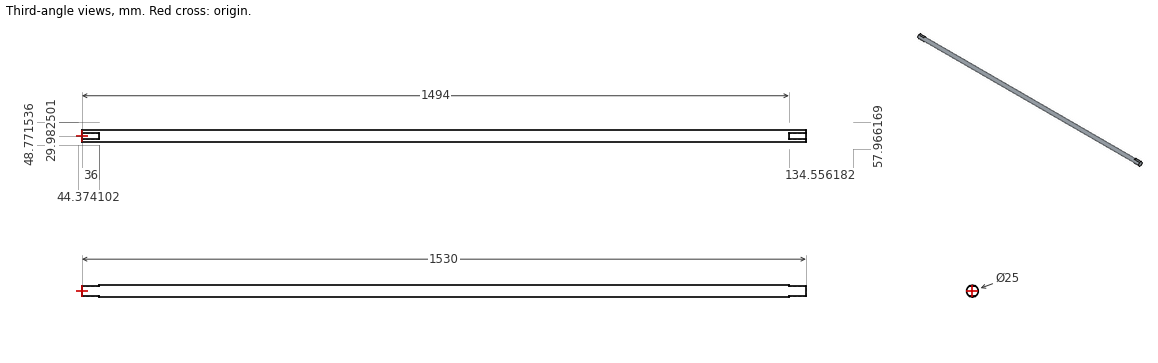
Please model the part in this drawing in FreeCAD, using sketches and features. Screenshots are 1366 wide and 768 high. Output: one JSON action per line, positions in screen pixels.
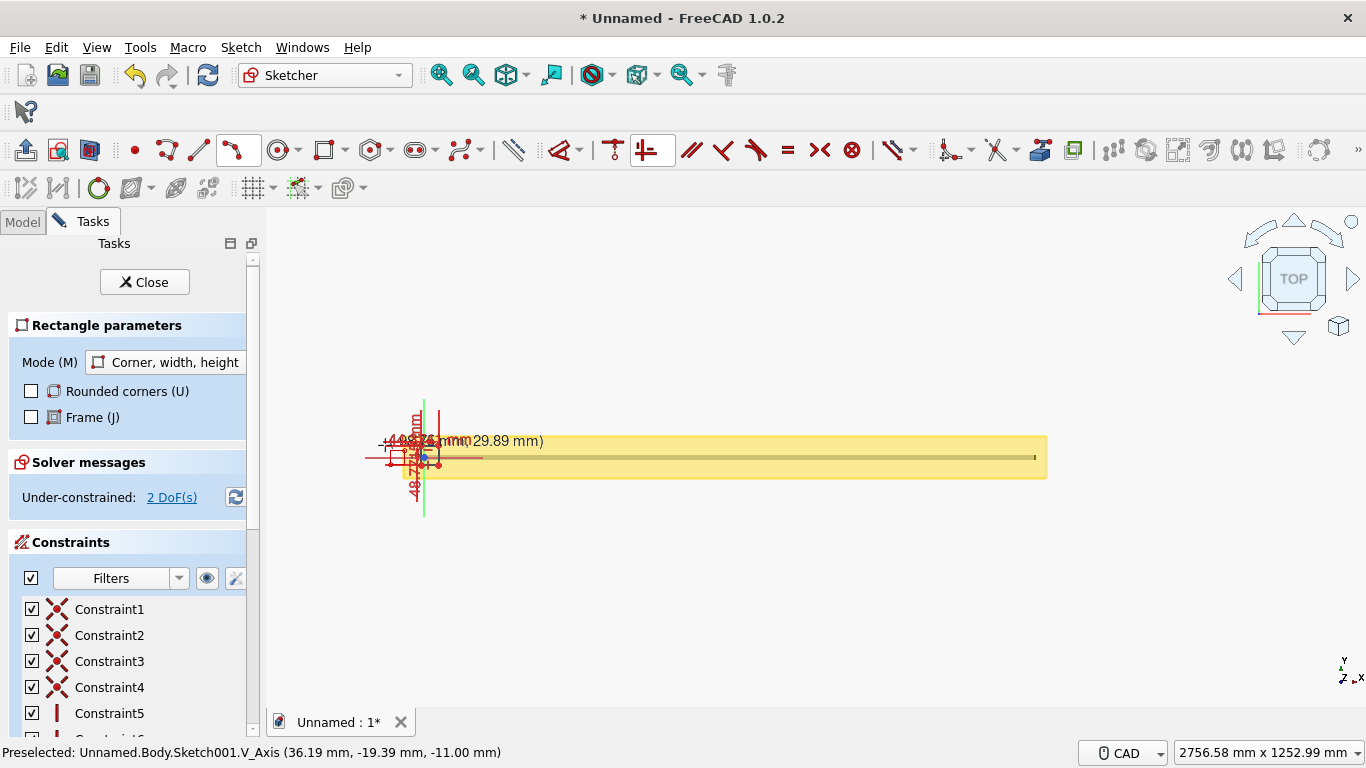
{"action": "scroll", "coordinate": [1021, 446], "scroll_direction": "up", "scroll_amount": 2}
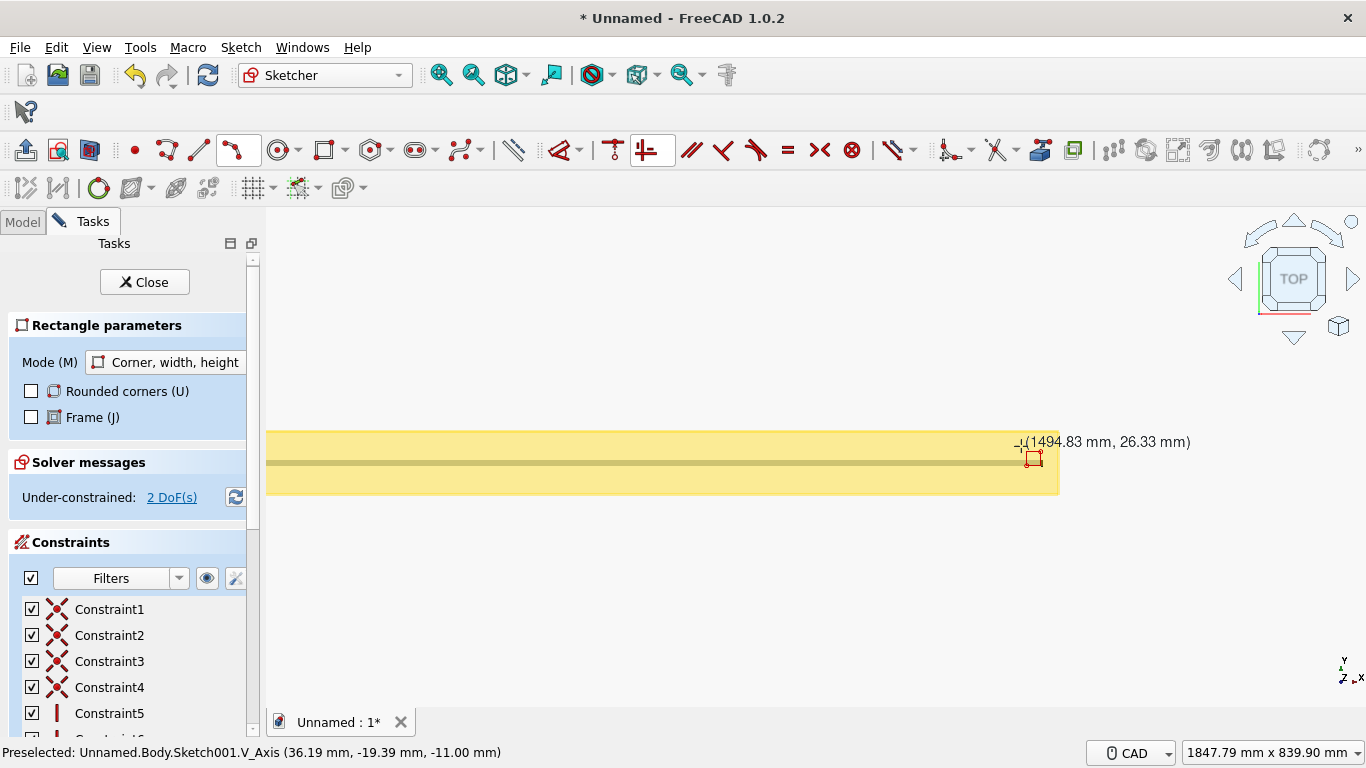
{"action": "left_click", "coordinate": [1020, 445]}
{"action": "mouse_move", "coordinate": [1100, 480]}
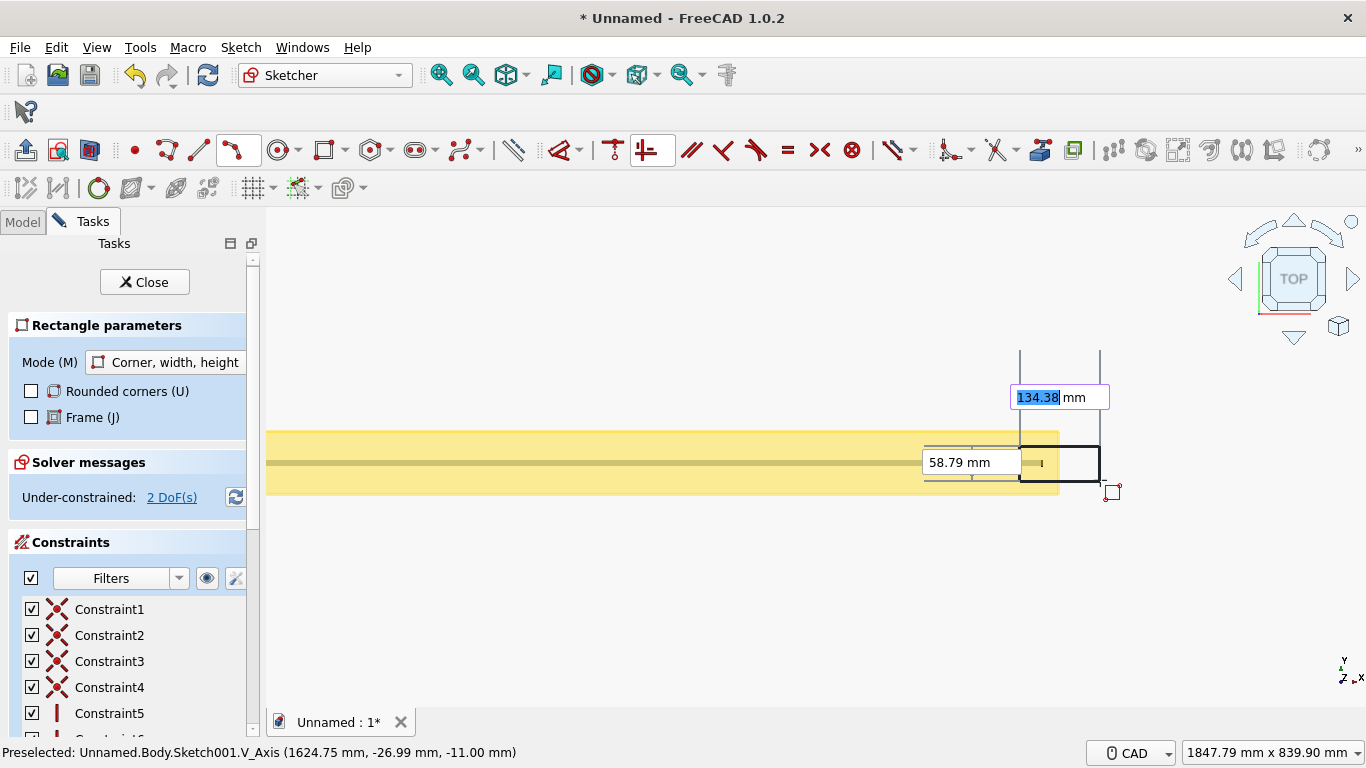
{"action": "type", "text": "134.556182"}
{"action": "key", "text": "Tab"}
{"action": "type", "text": "57.966169"}
{"action": "key", "text": "Return"}
{"action": "key", "text": "Escape"}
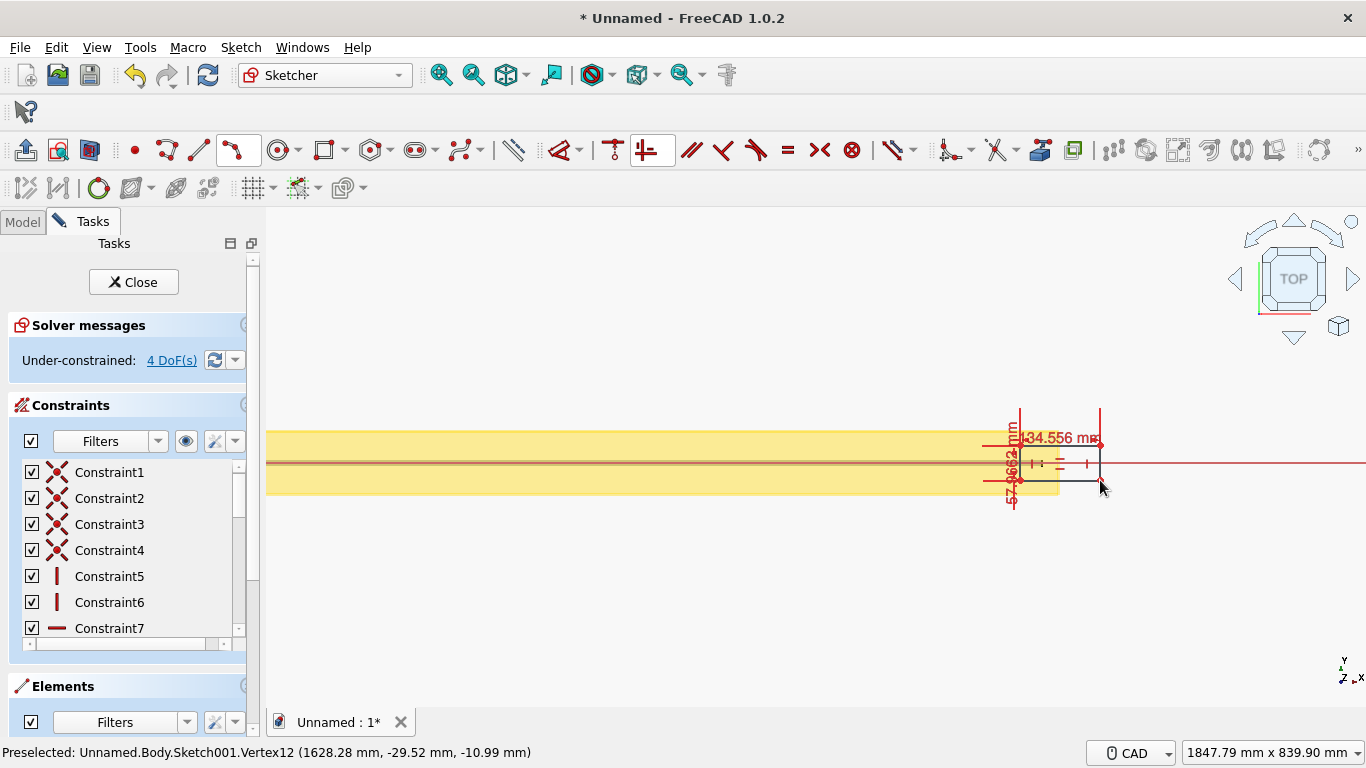
{"action": "left_click", "coordinate": [560, 150]}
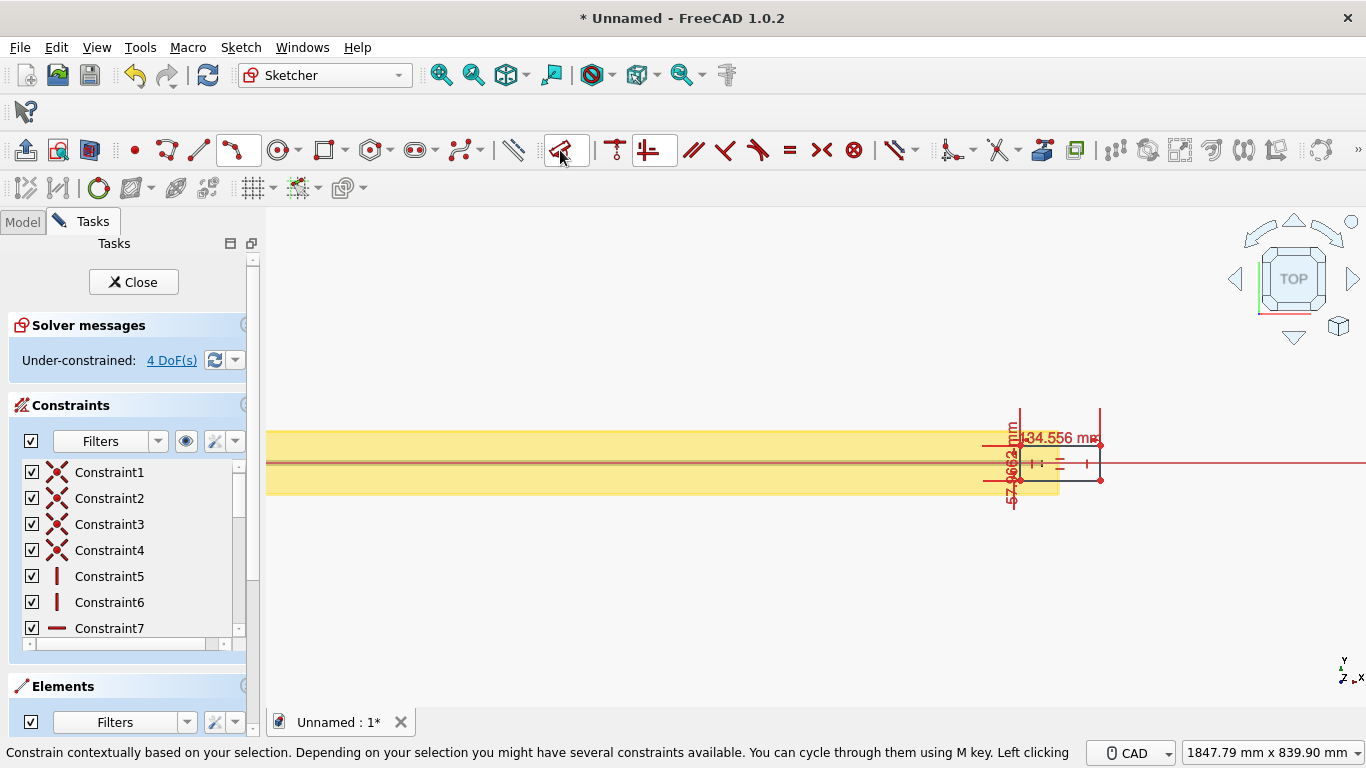
{"action": "scroll", "coordinate": [1021, 446], "scroll_direction": "down", "scroll_amount": 2}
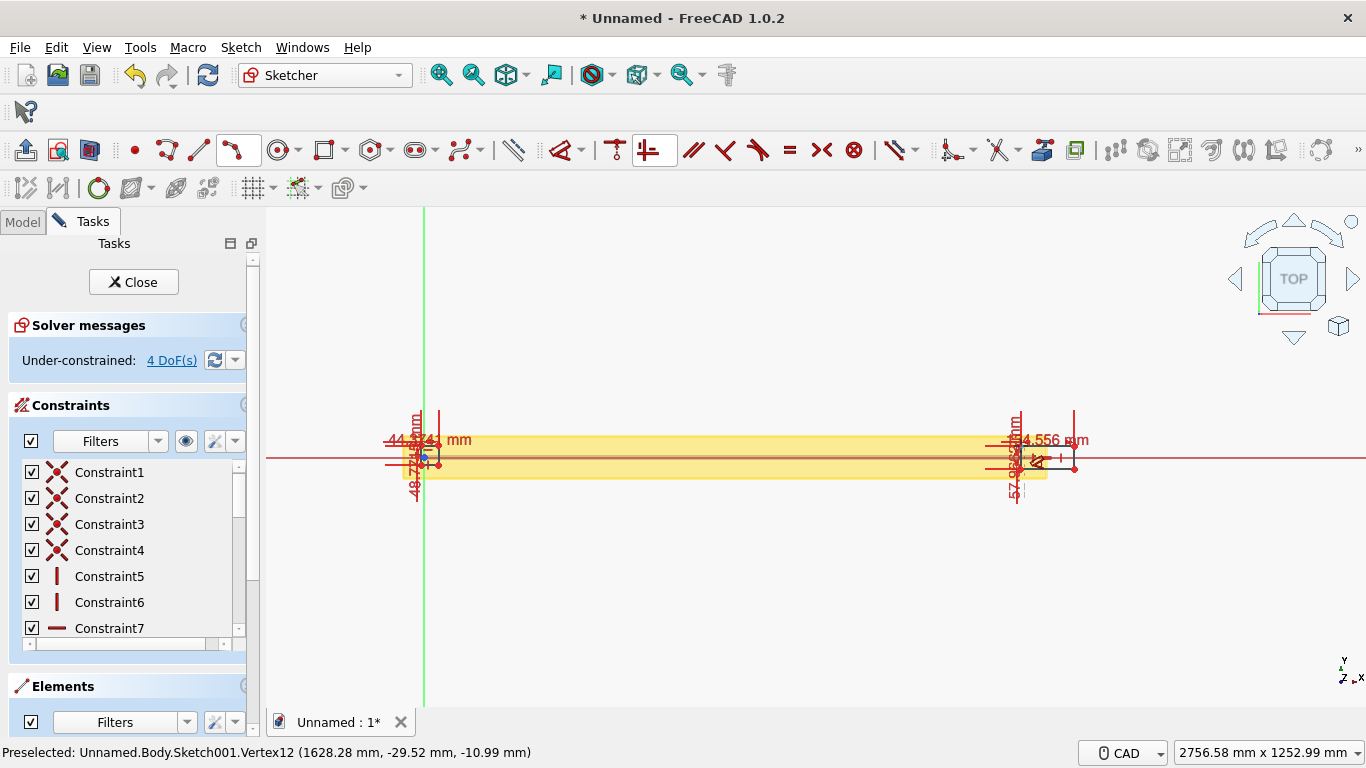
{"action": "scroll", "coordinate": [439, 465], "scroll_direction": "up", "scroll_amount": 6}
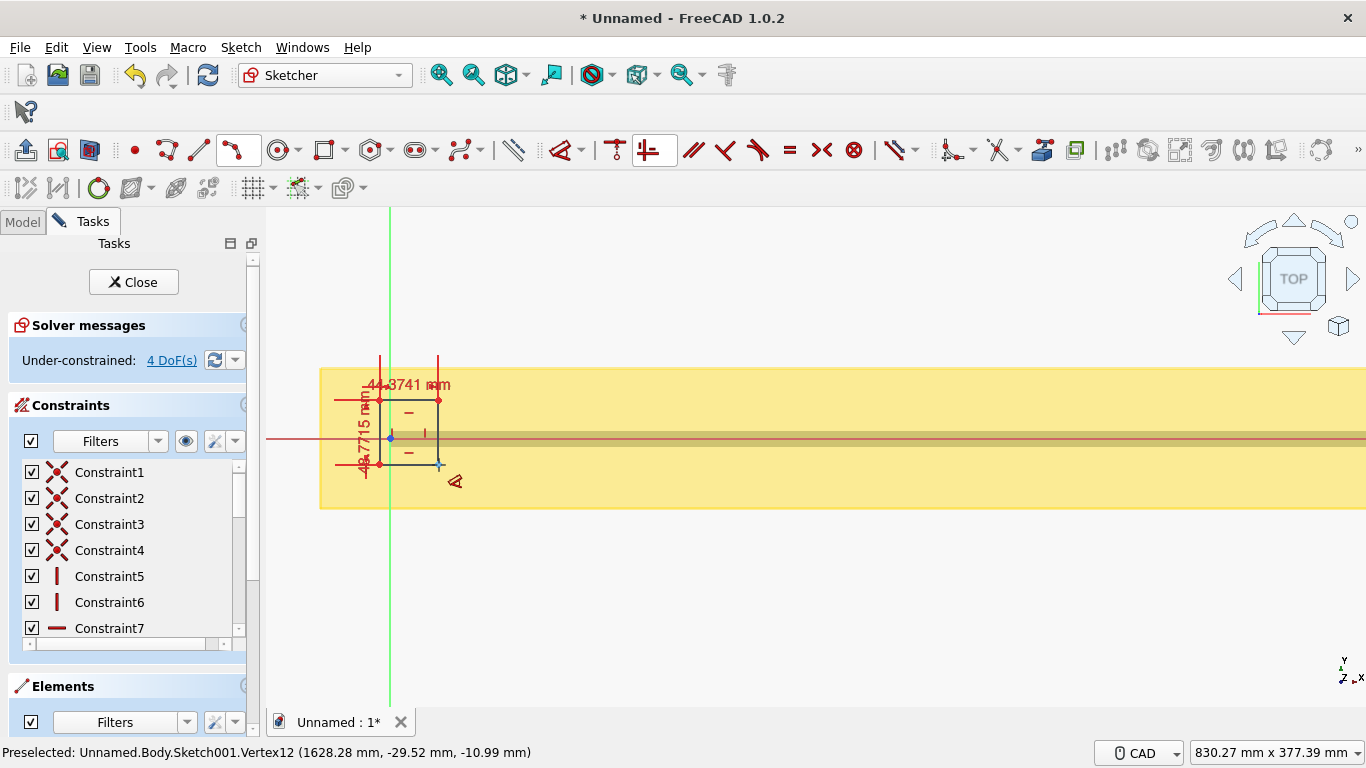
{"action": "left_click", "coordinate": [438, 465]}
{"action": "left_click", "coordinate": [414, 499]}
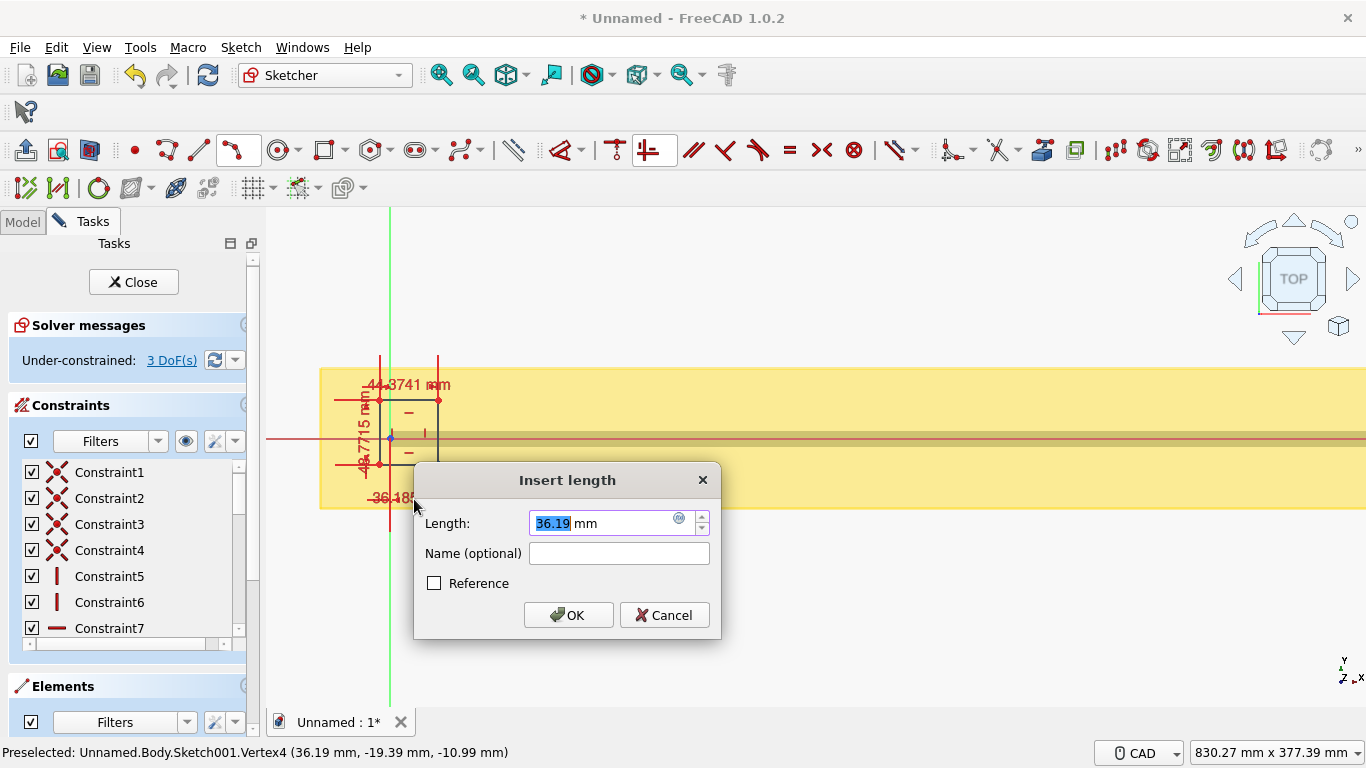
{"action": "type", "text": "36"}
{"action": "key", "text": "Return"}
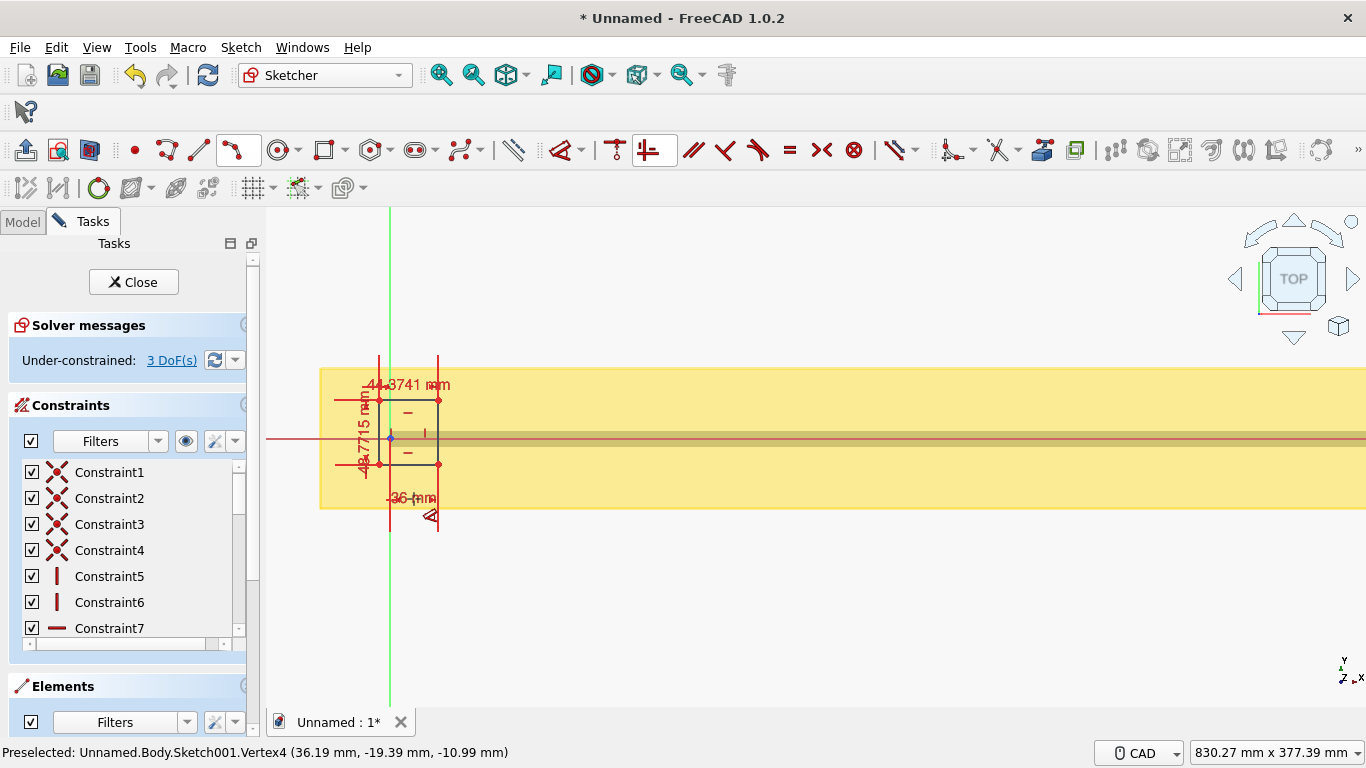
{"action": "scroll", "coordinate": [439, 465], "scroll_direction": "down", "scroll_amount": 6}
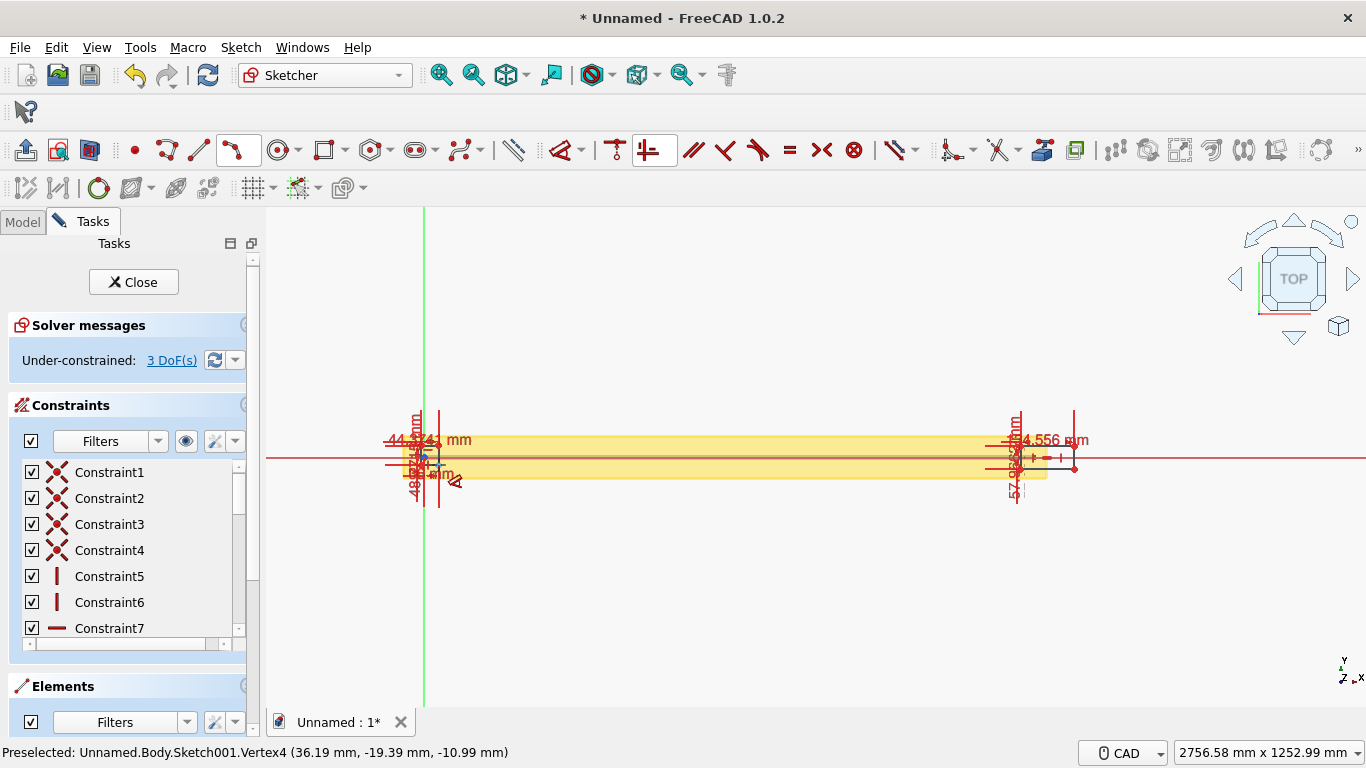
{"action": "left_click", "coordinate": [1021, 446]}
{"action": "left_click", "coordinate": [723, 412]}